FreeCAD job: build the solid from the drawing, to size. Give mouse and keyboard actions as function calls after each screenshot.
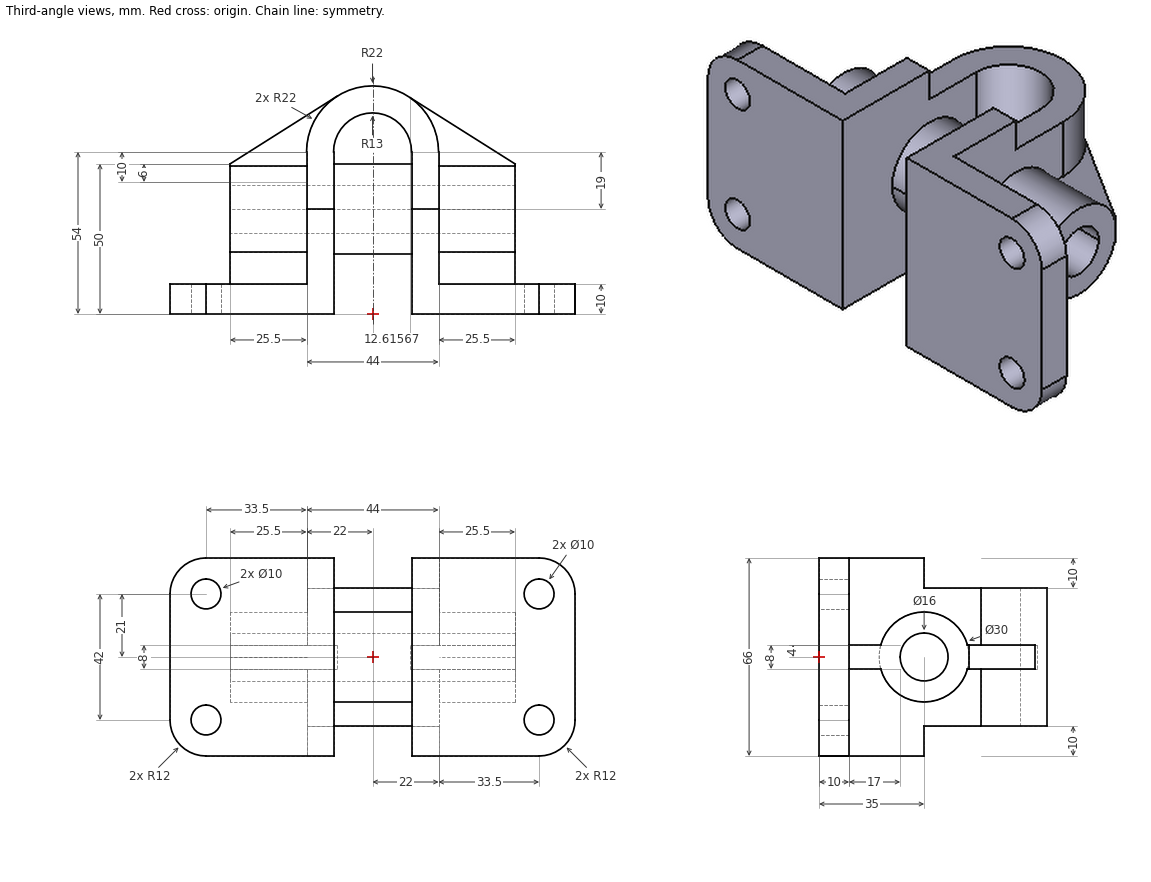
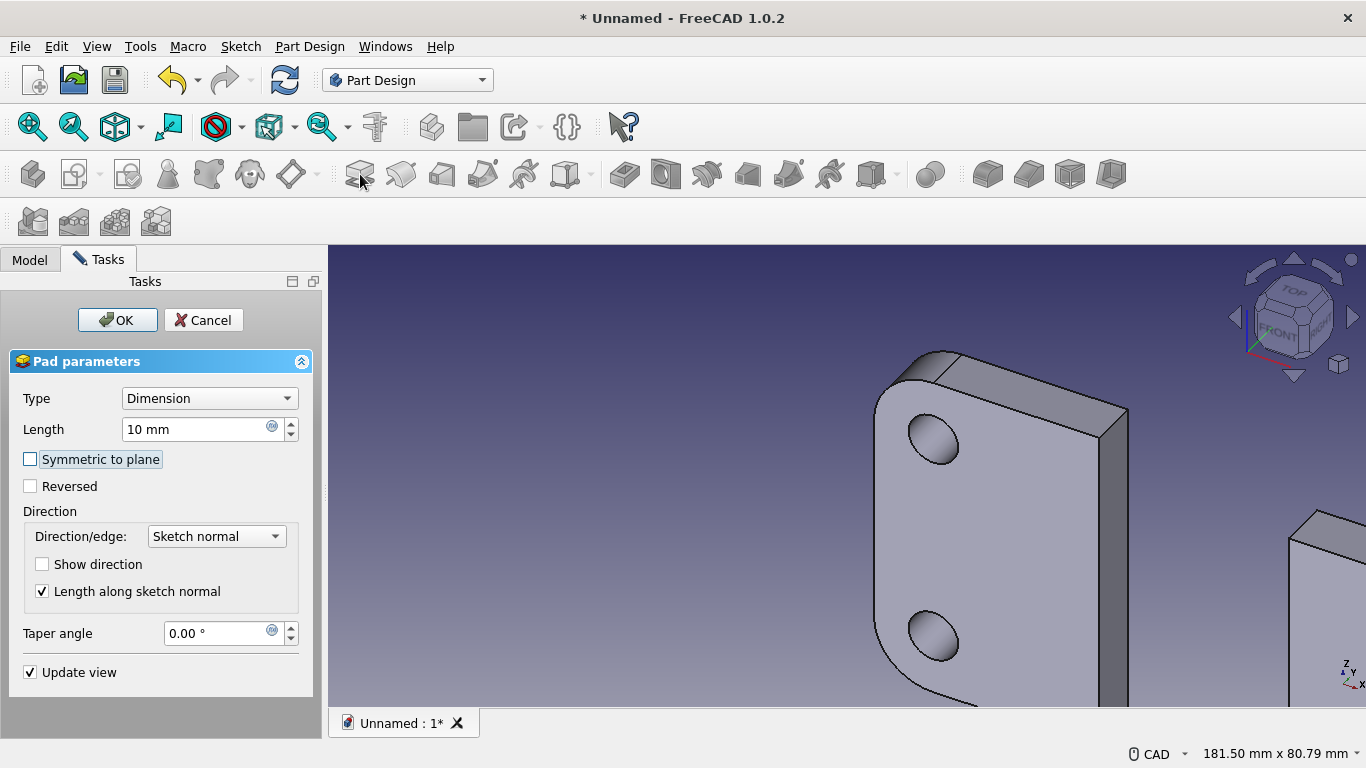
click(31, 486)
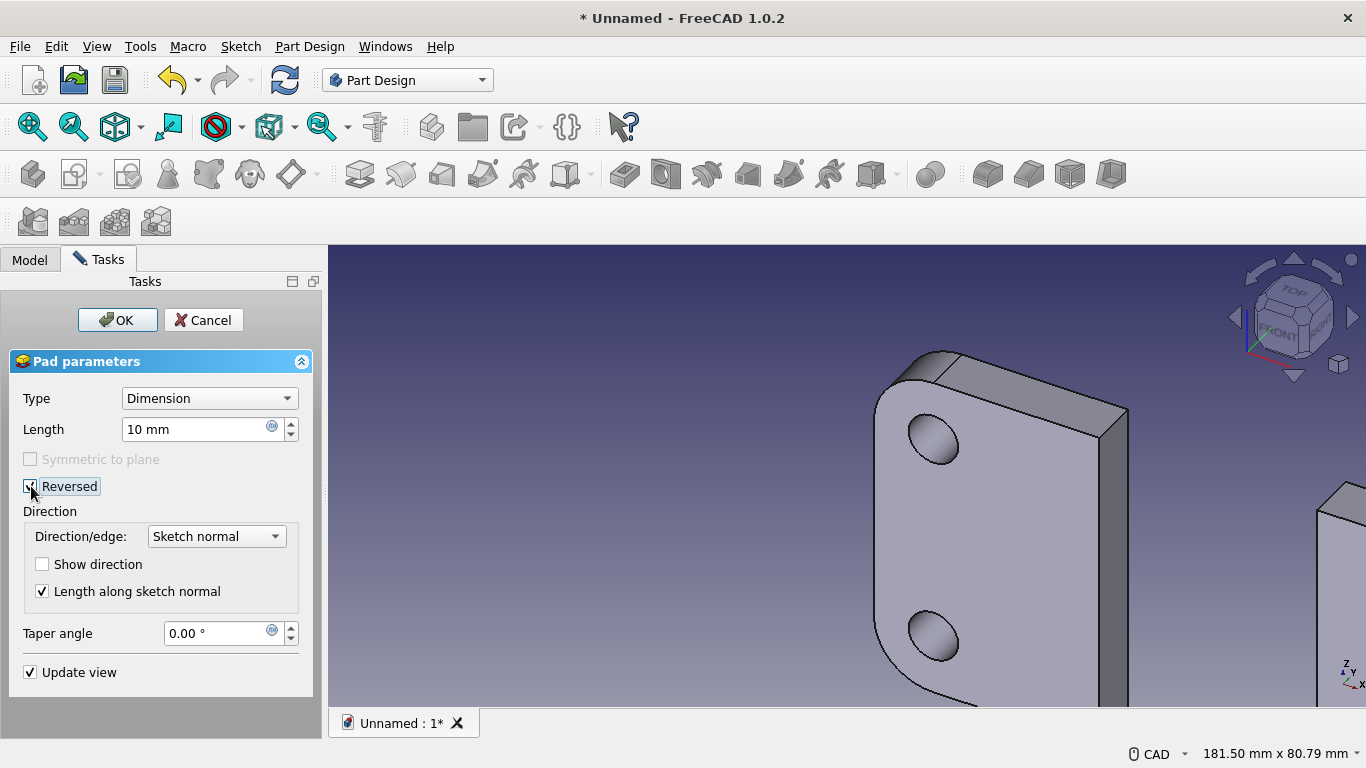
click(118, 320)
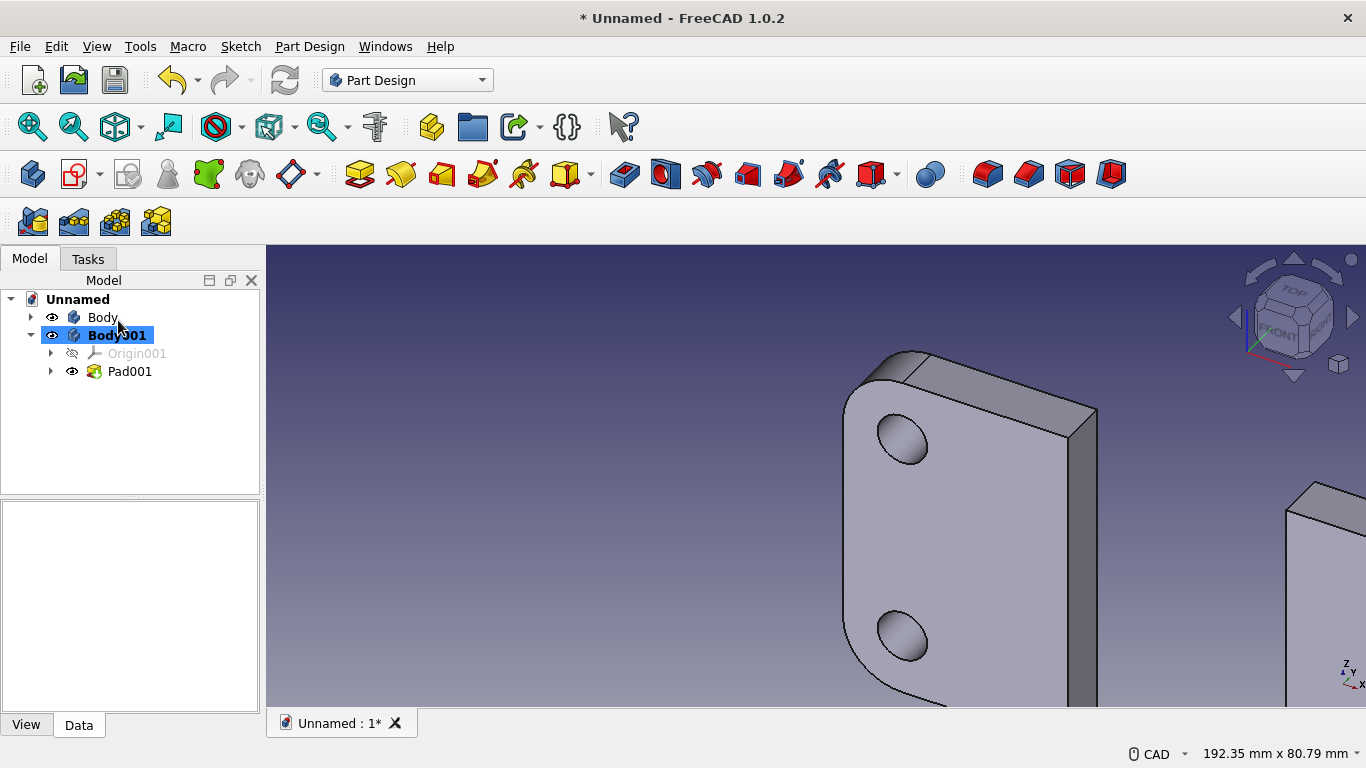
click(33, 128)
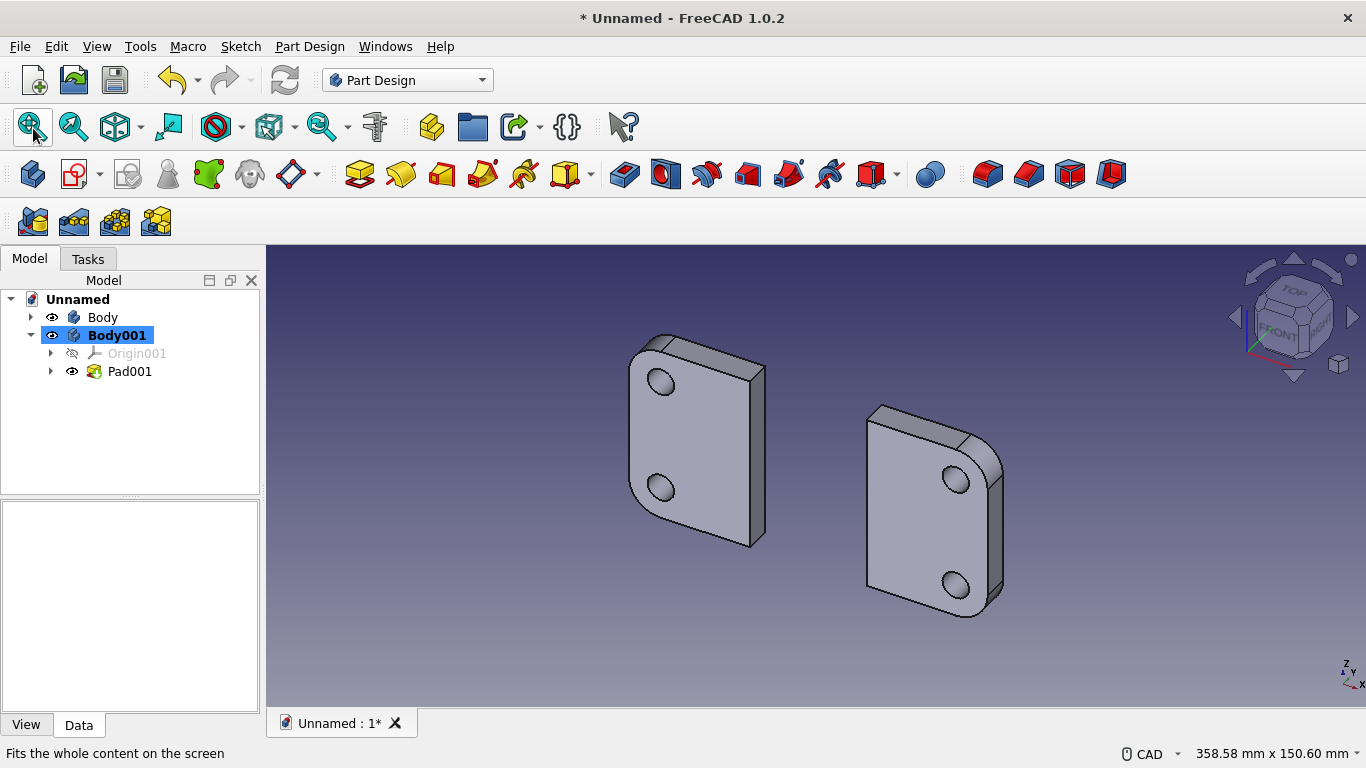
double_click(97, 317)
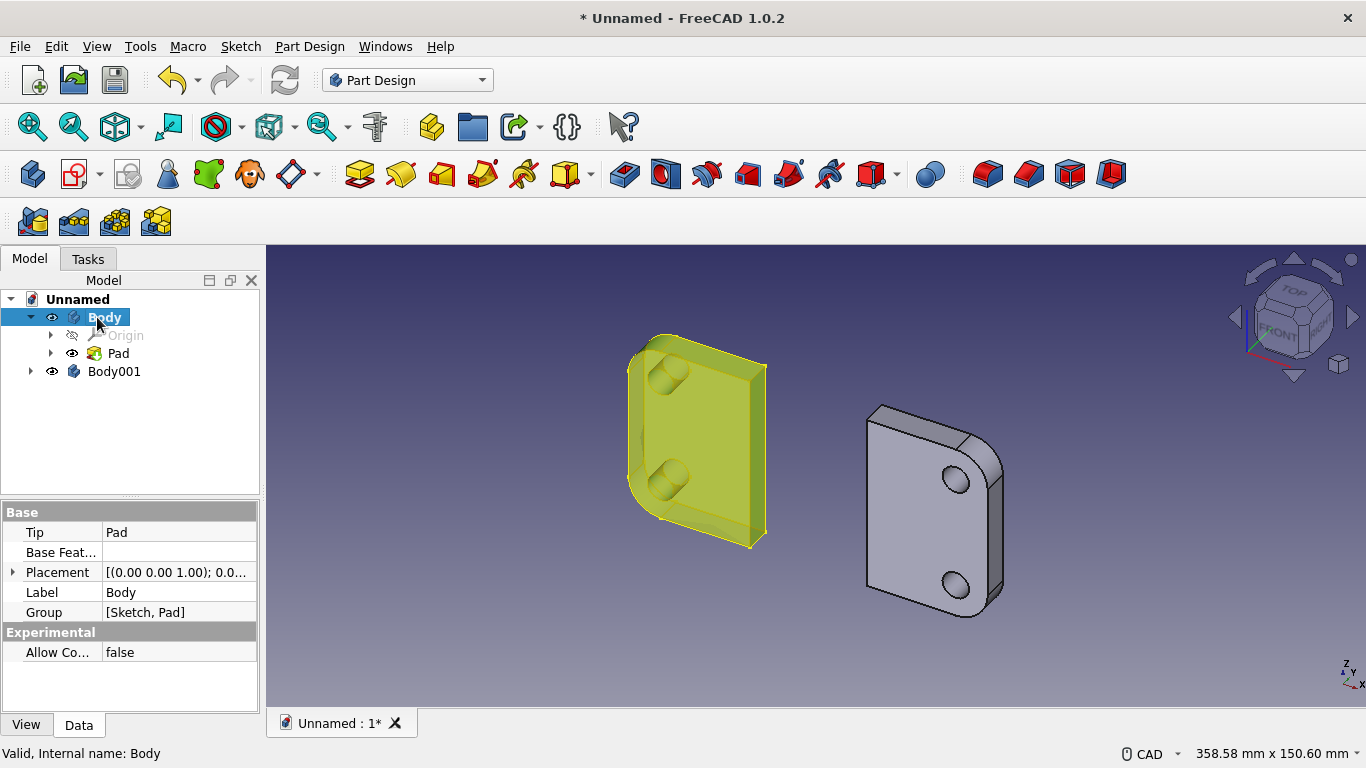
click(97, 317)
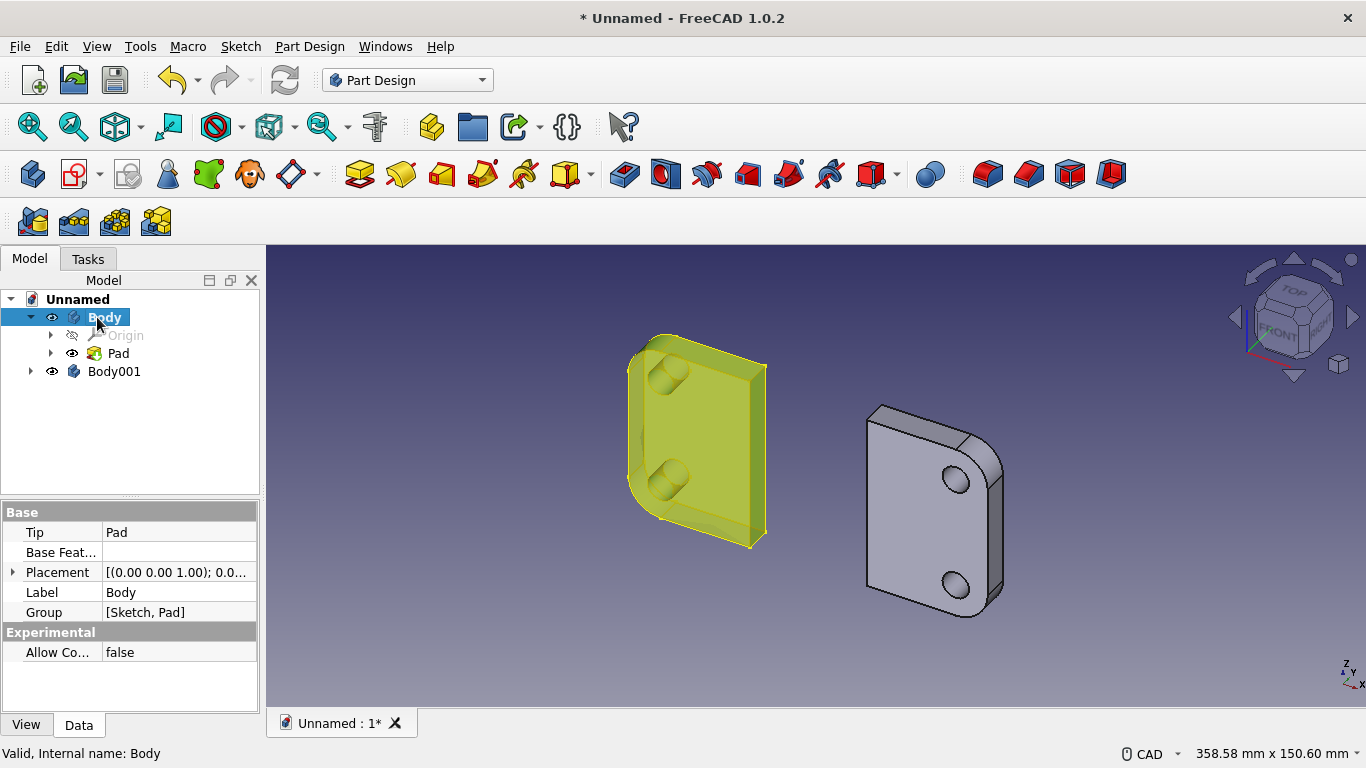
click(148, 652)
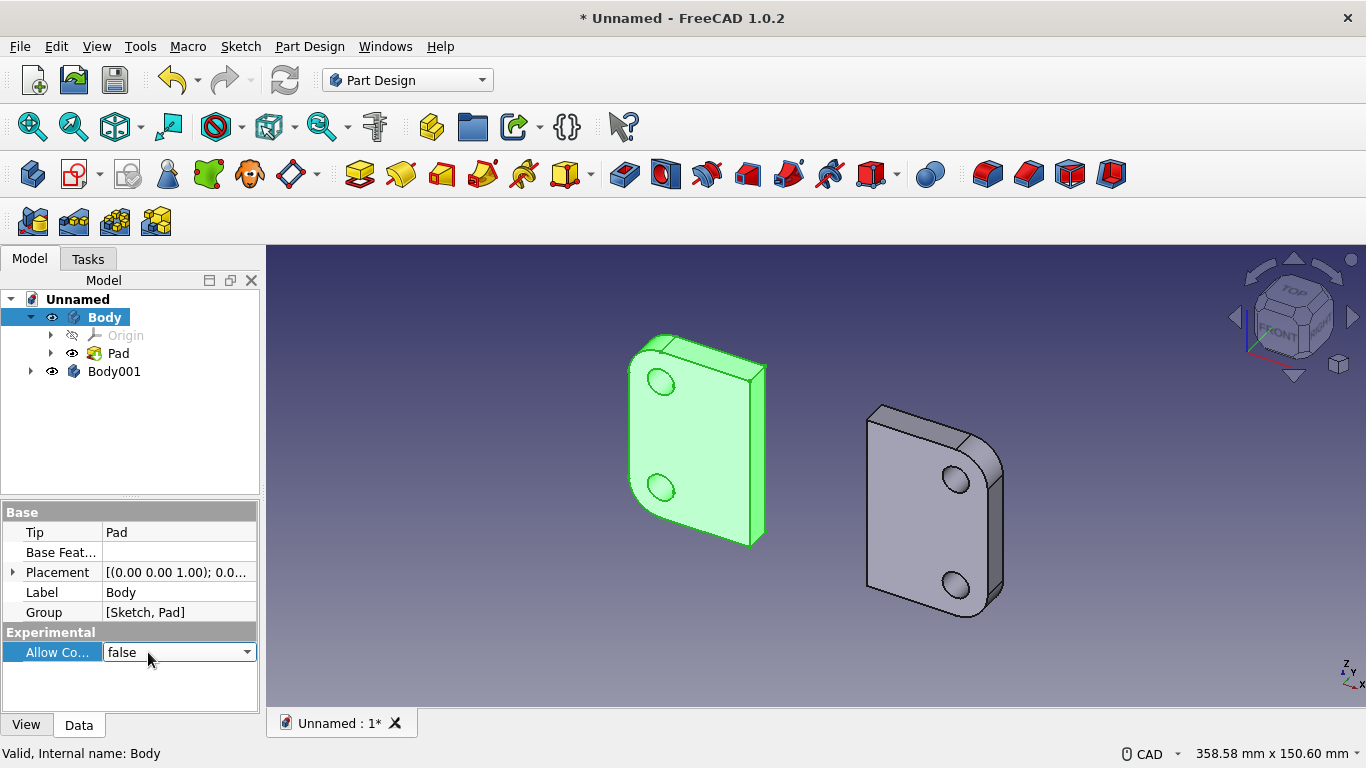
click(148, 652)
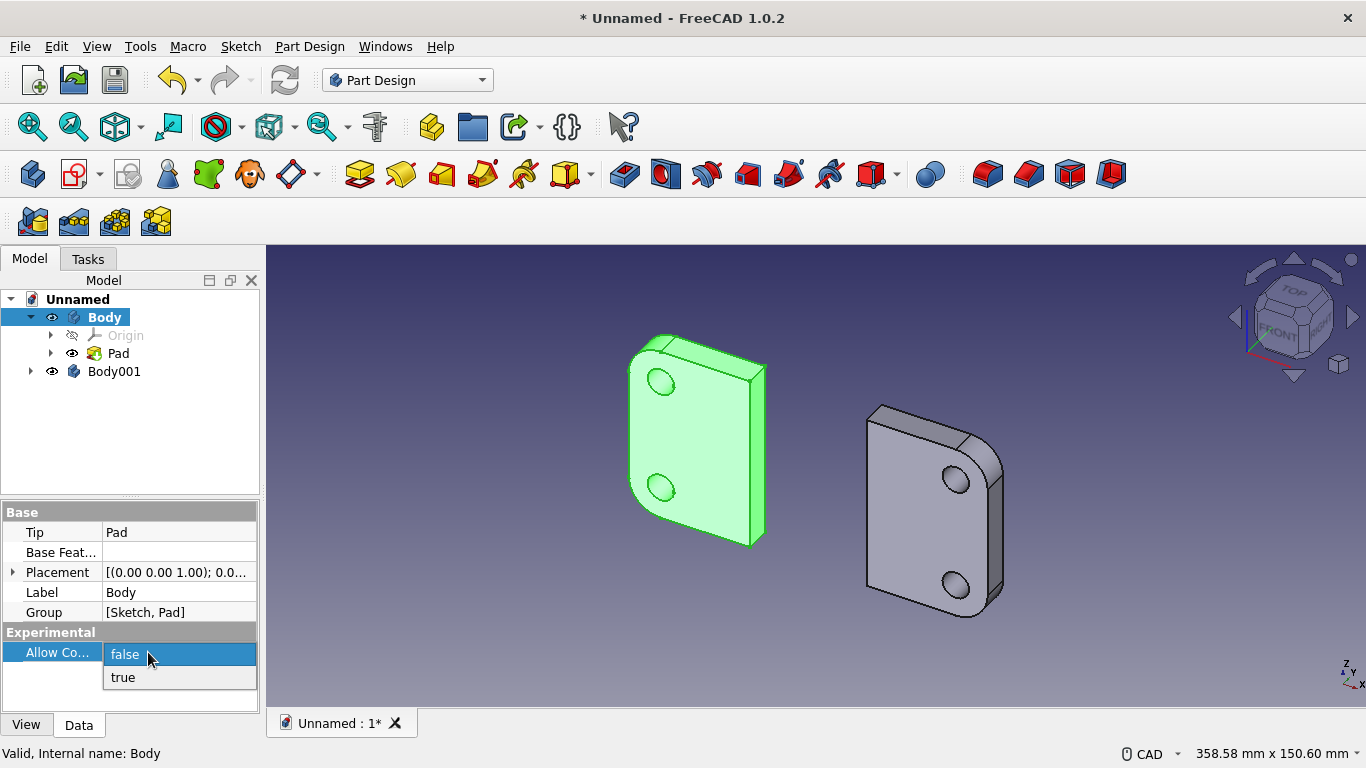
click(178, 678)
key(Return)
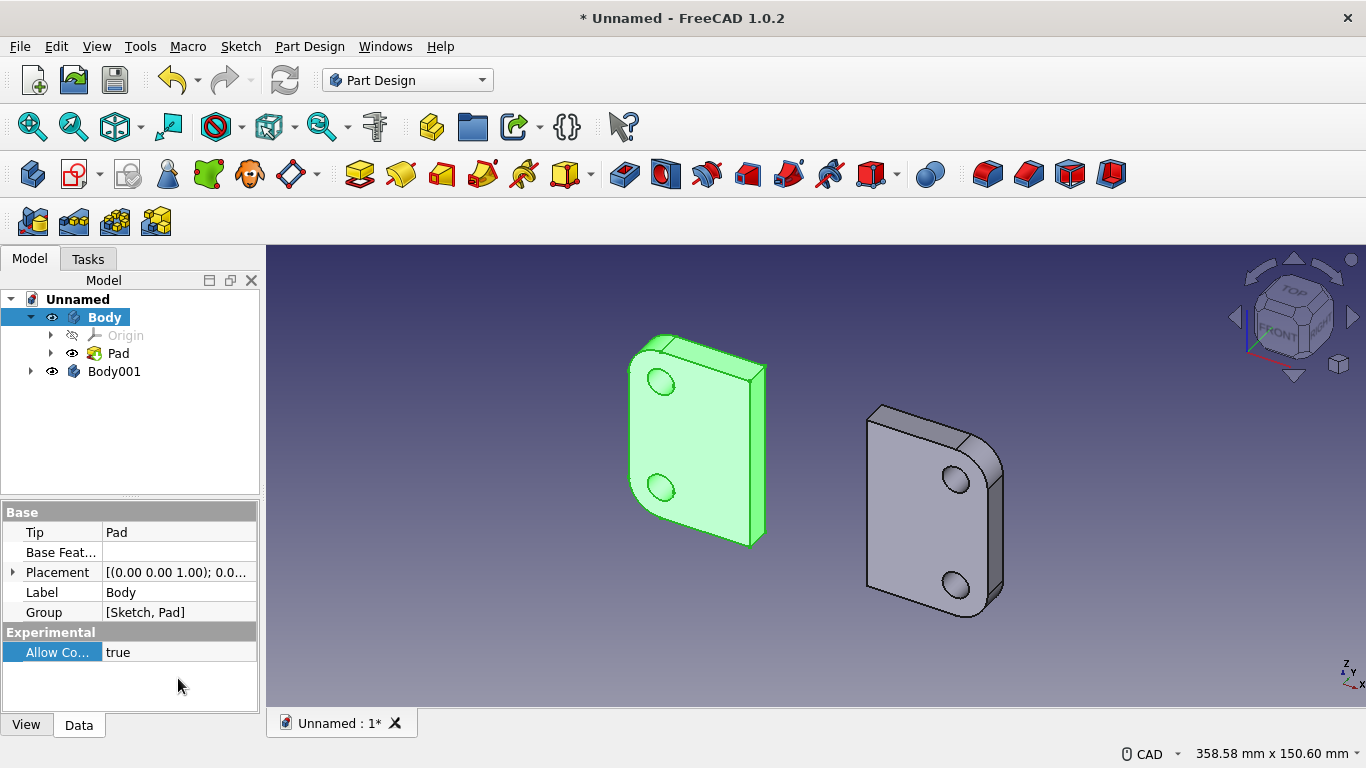
click(97, 371)